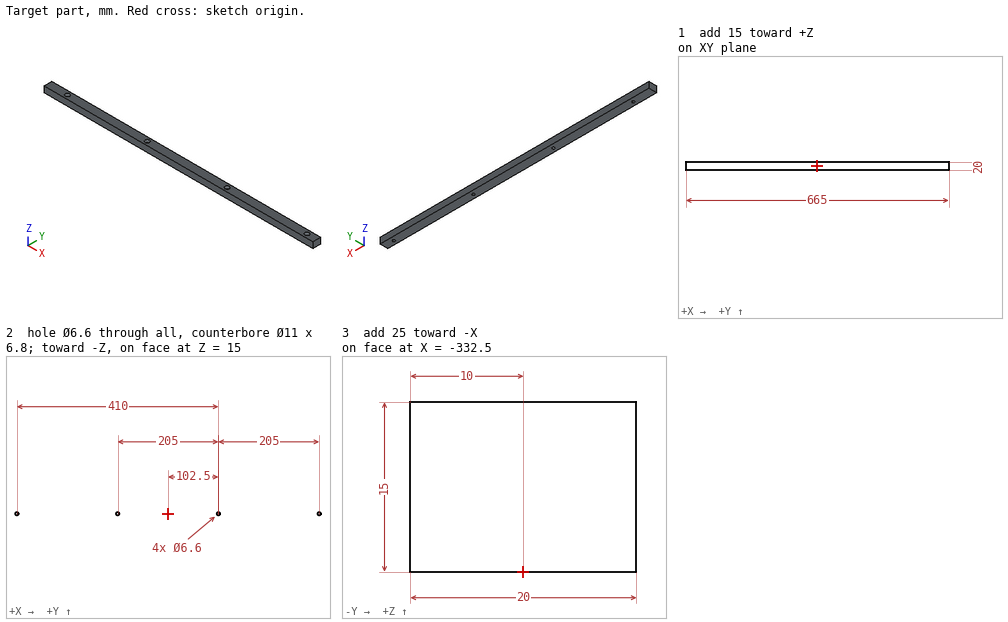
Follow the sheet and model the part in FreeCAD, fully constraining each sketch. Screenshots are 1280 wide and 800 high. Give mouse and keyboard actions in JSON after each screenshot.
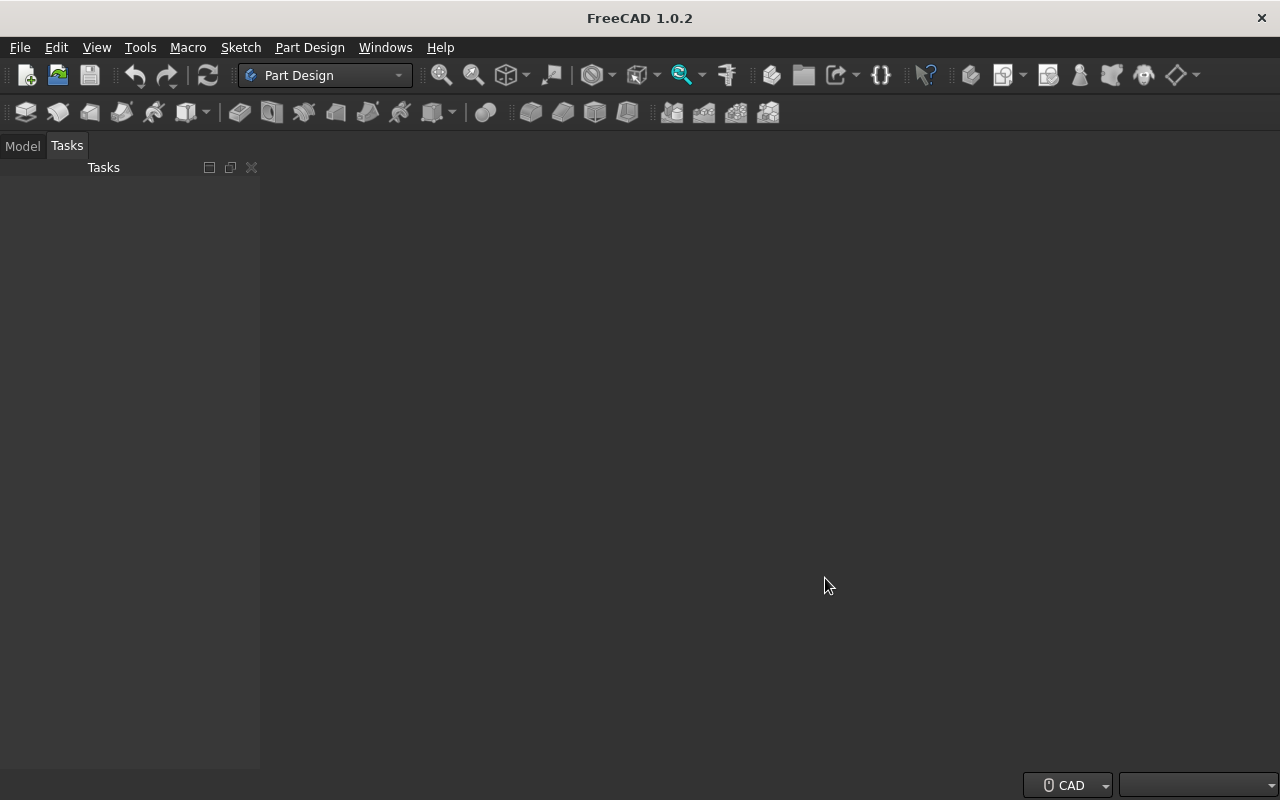
{"action": "key", "text": "ctrl+n"}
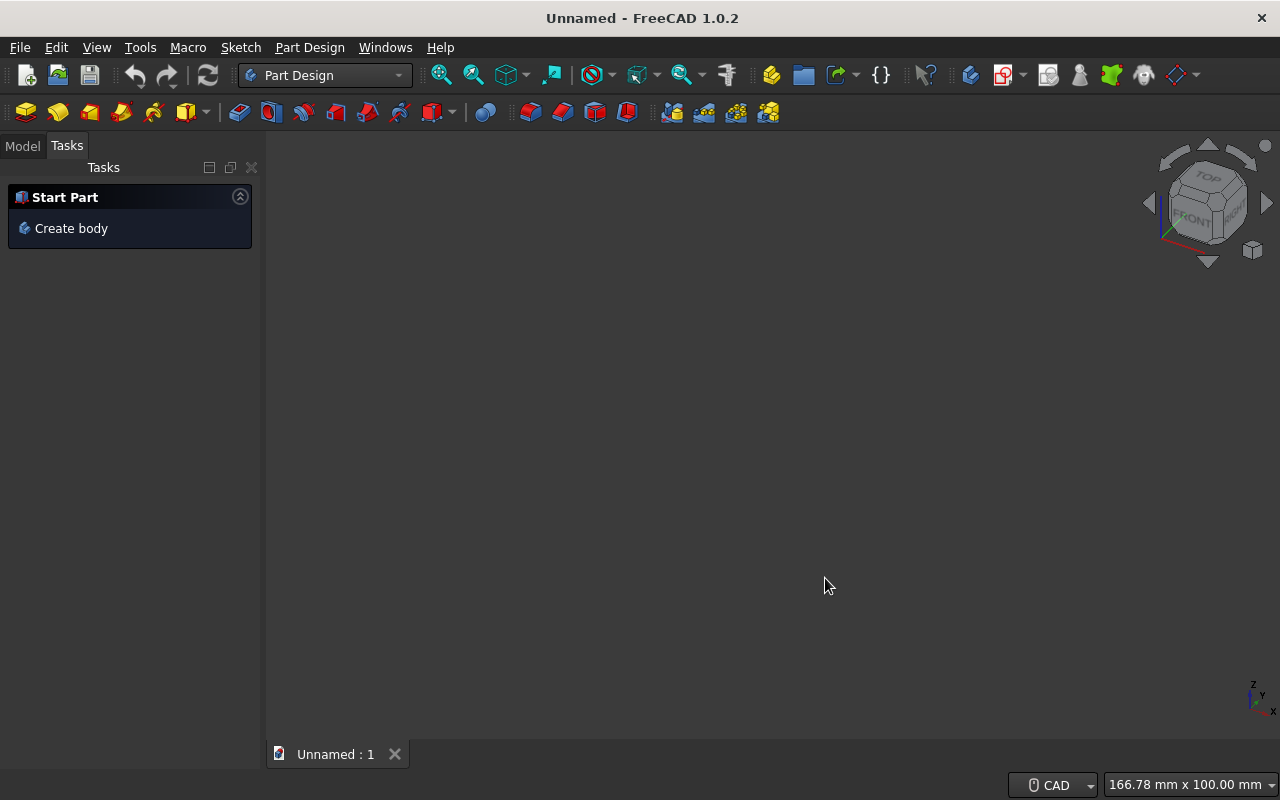
{"action": "left_click", "coordinate": [1004, 76]}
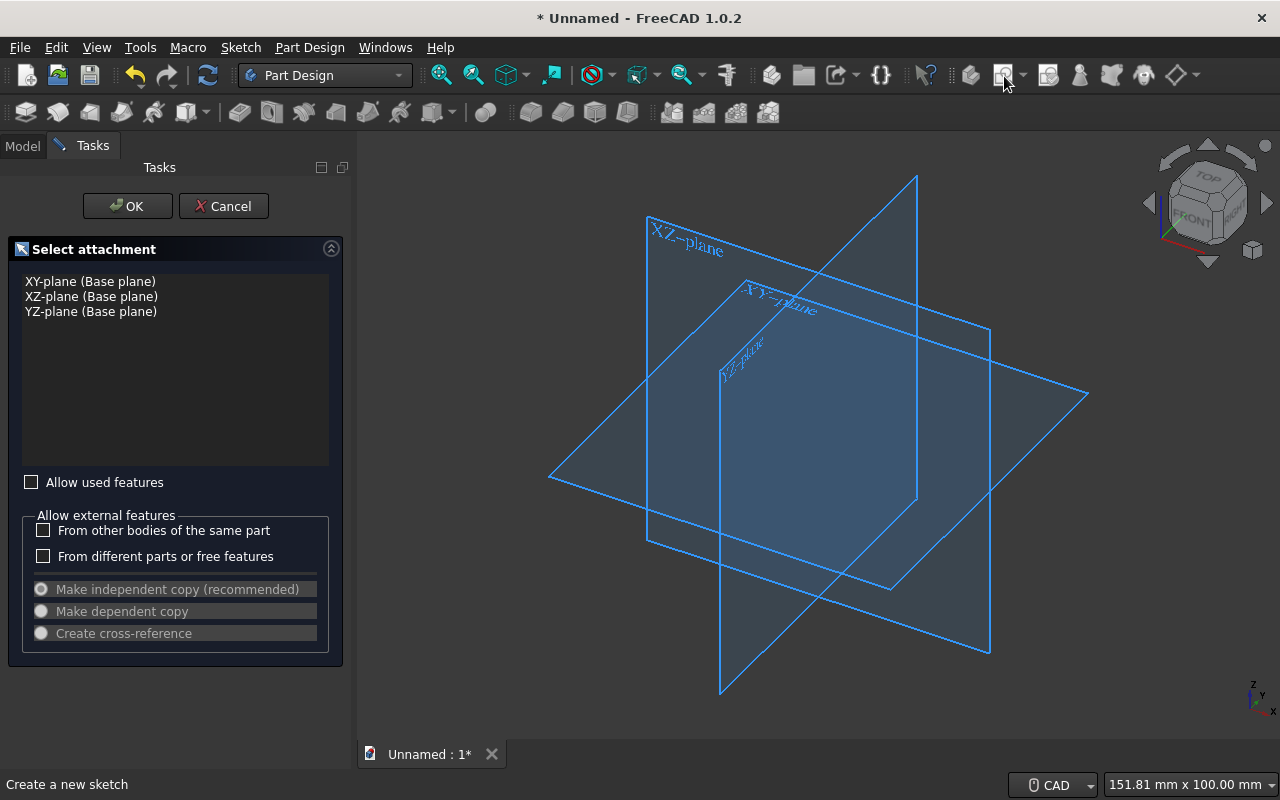
{"action": "left_click", "coordinate": [82, 282]}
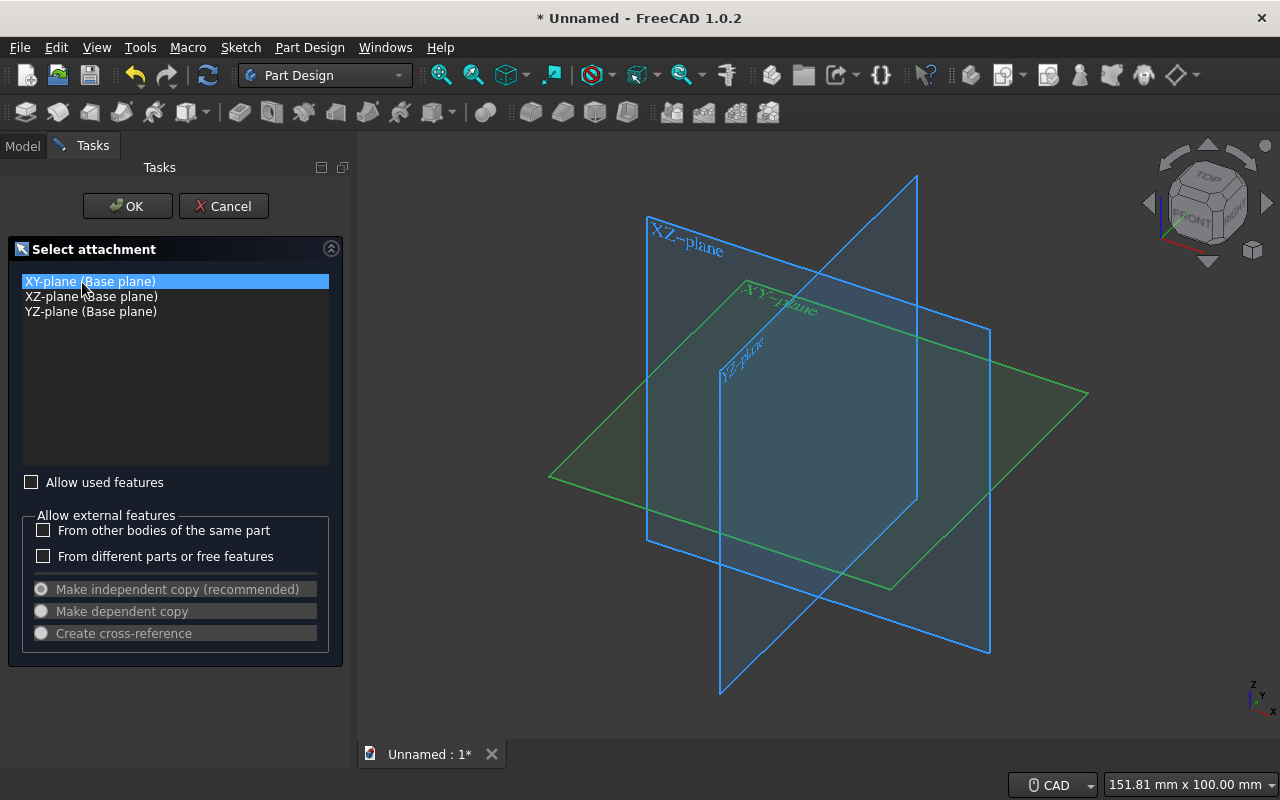
{"action": "left_click", "coordinate": [128, 206]}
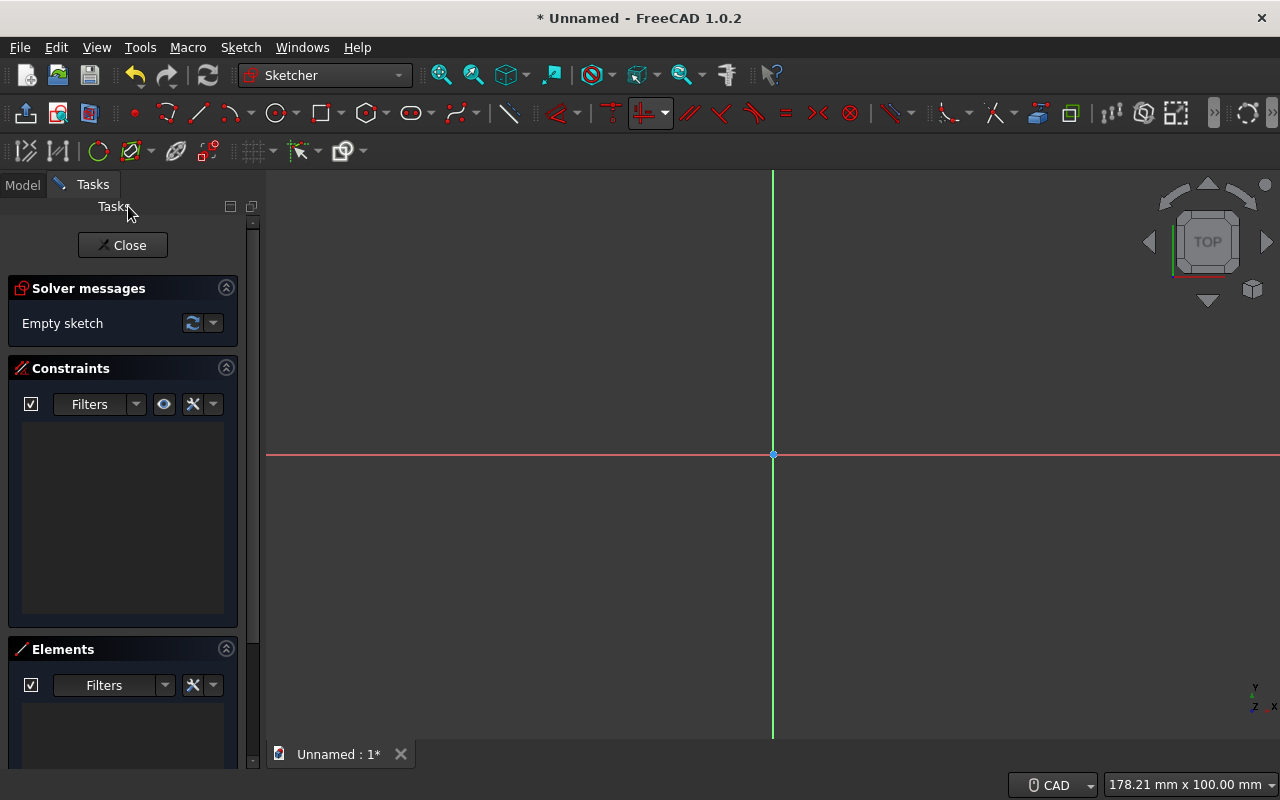
{"action": "scroll", "coordinate": [691, 454], "scroll_direction": "down", "scroll_amount": 9}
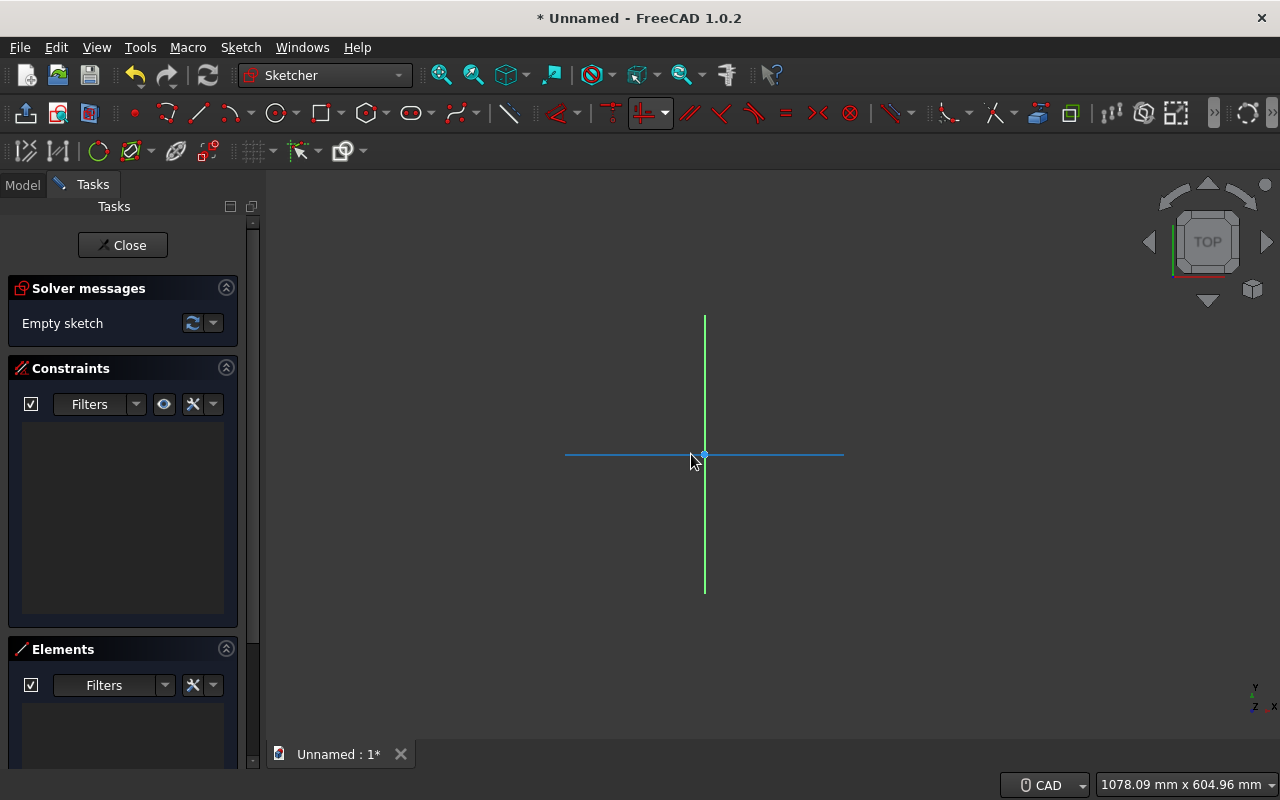
{"action": "key", "text": "g v"}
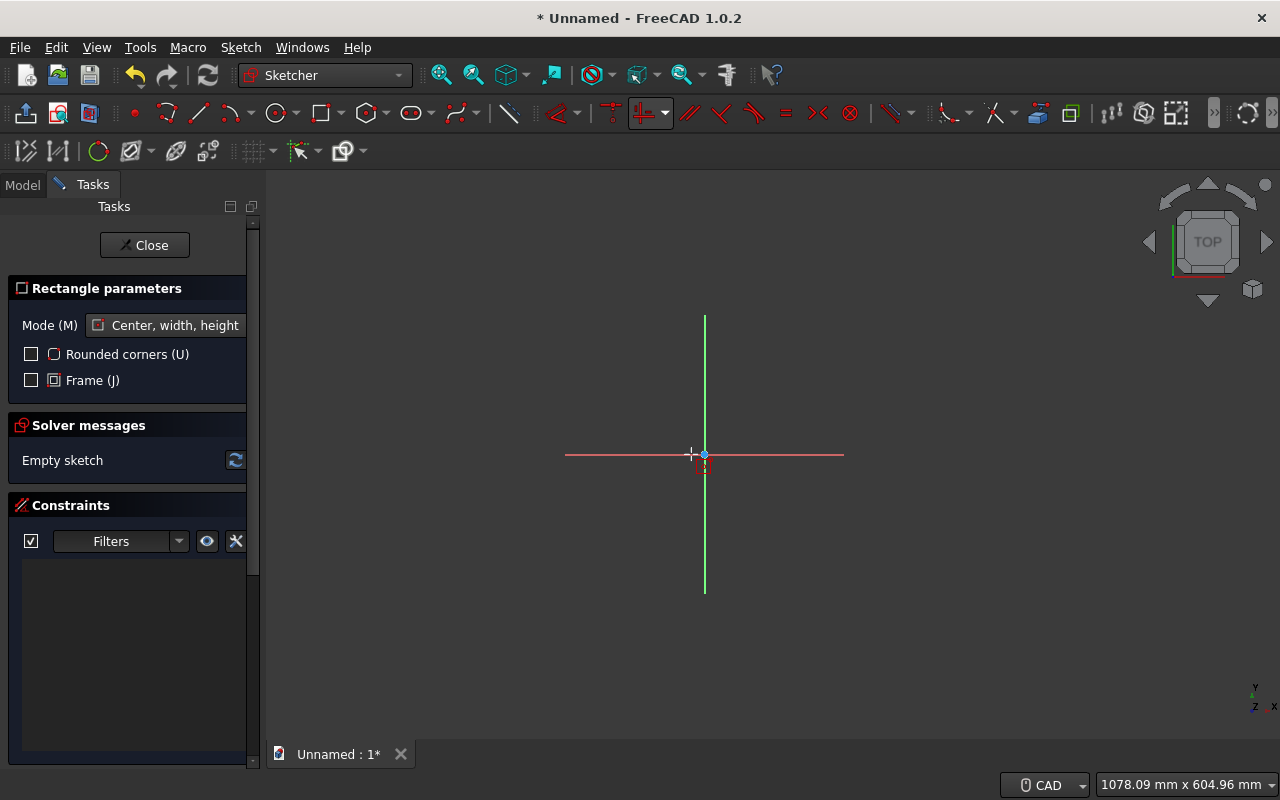
{"action": "scroll", "coordinate": [705, 454], "scroll_direction": "up", "scroll_amount": 3}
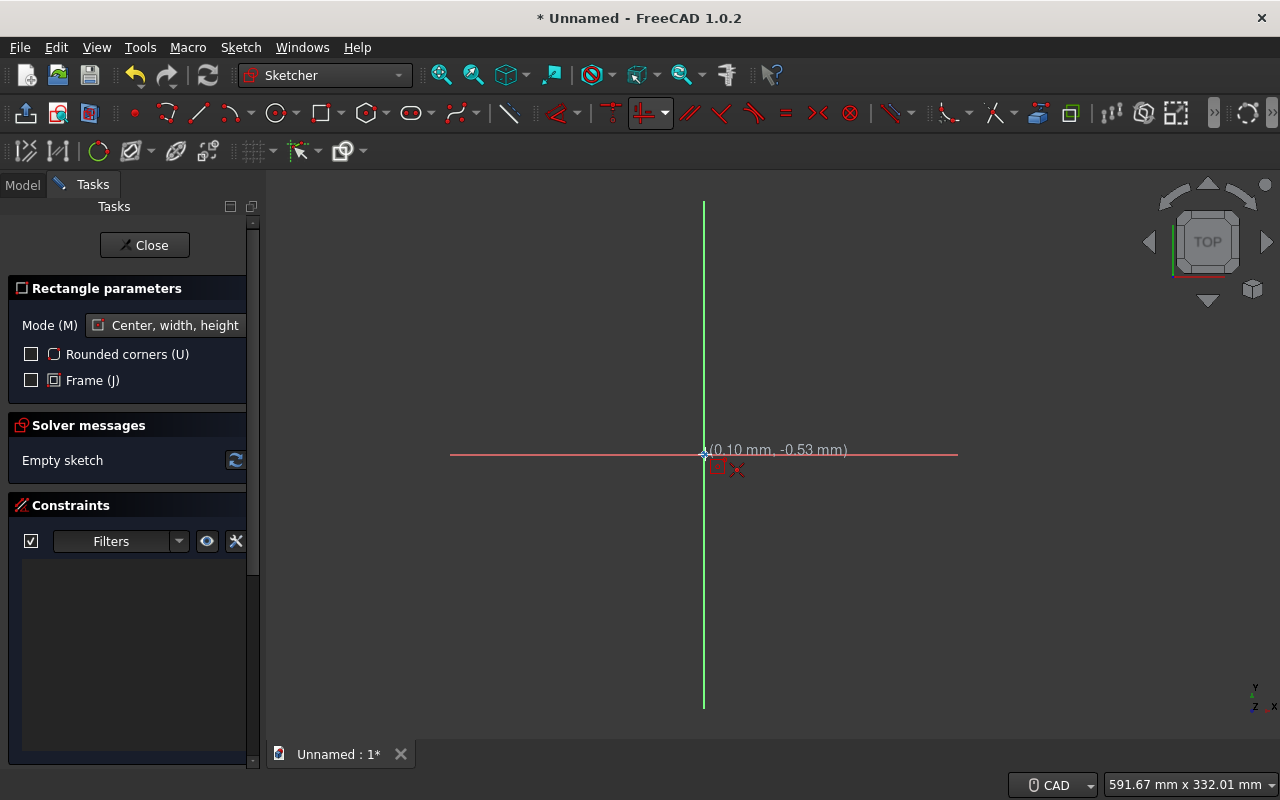
{"action": "left_click", "coordinate": [704, 454]}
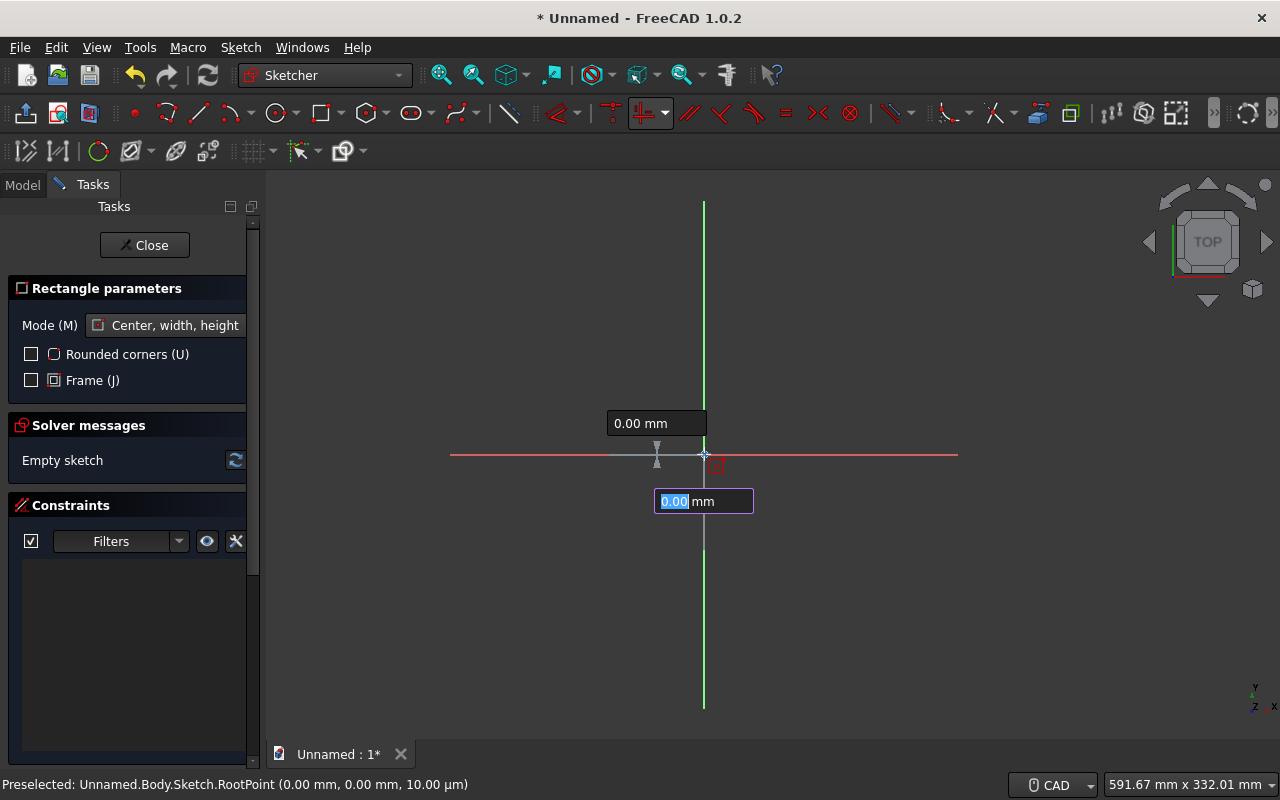
{"action": "scroll", "coordinate": [705, 454], "scroll_direction": "down", "scroll_amount": 3}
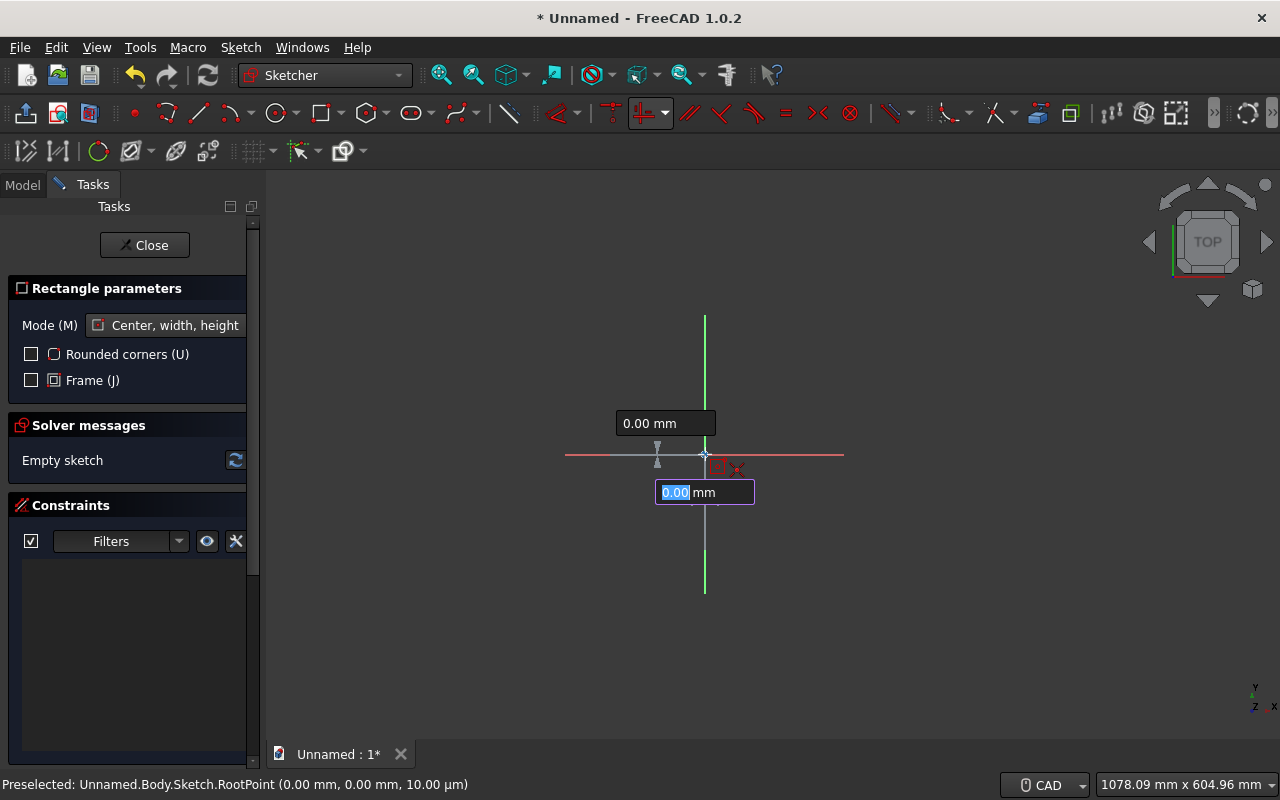
{"action": "scroll", "coordinate": [1018, 445], "scroll_direction": "up", "scroll_amount": 3}